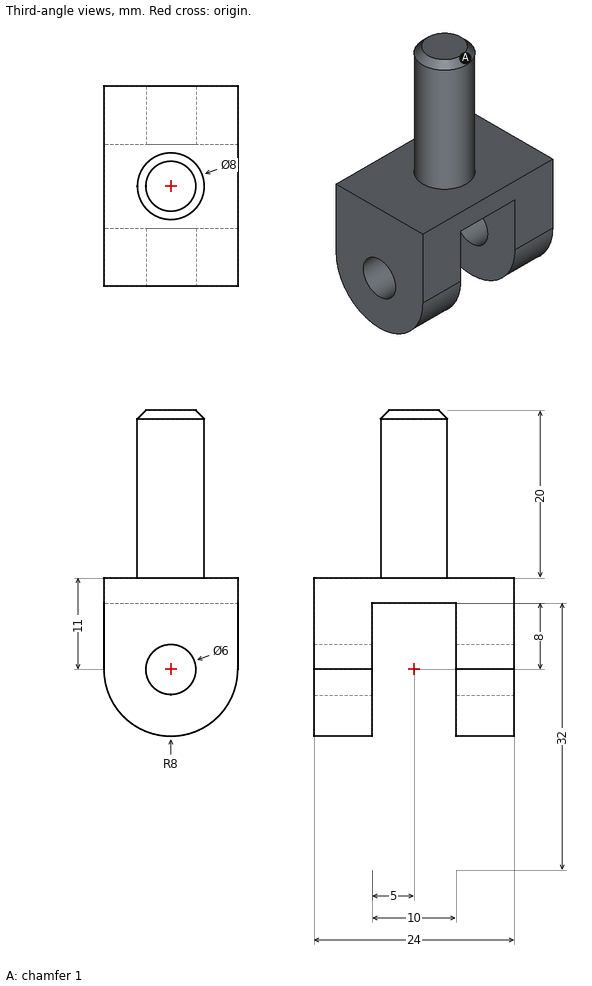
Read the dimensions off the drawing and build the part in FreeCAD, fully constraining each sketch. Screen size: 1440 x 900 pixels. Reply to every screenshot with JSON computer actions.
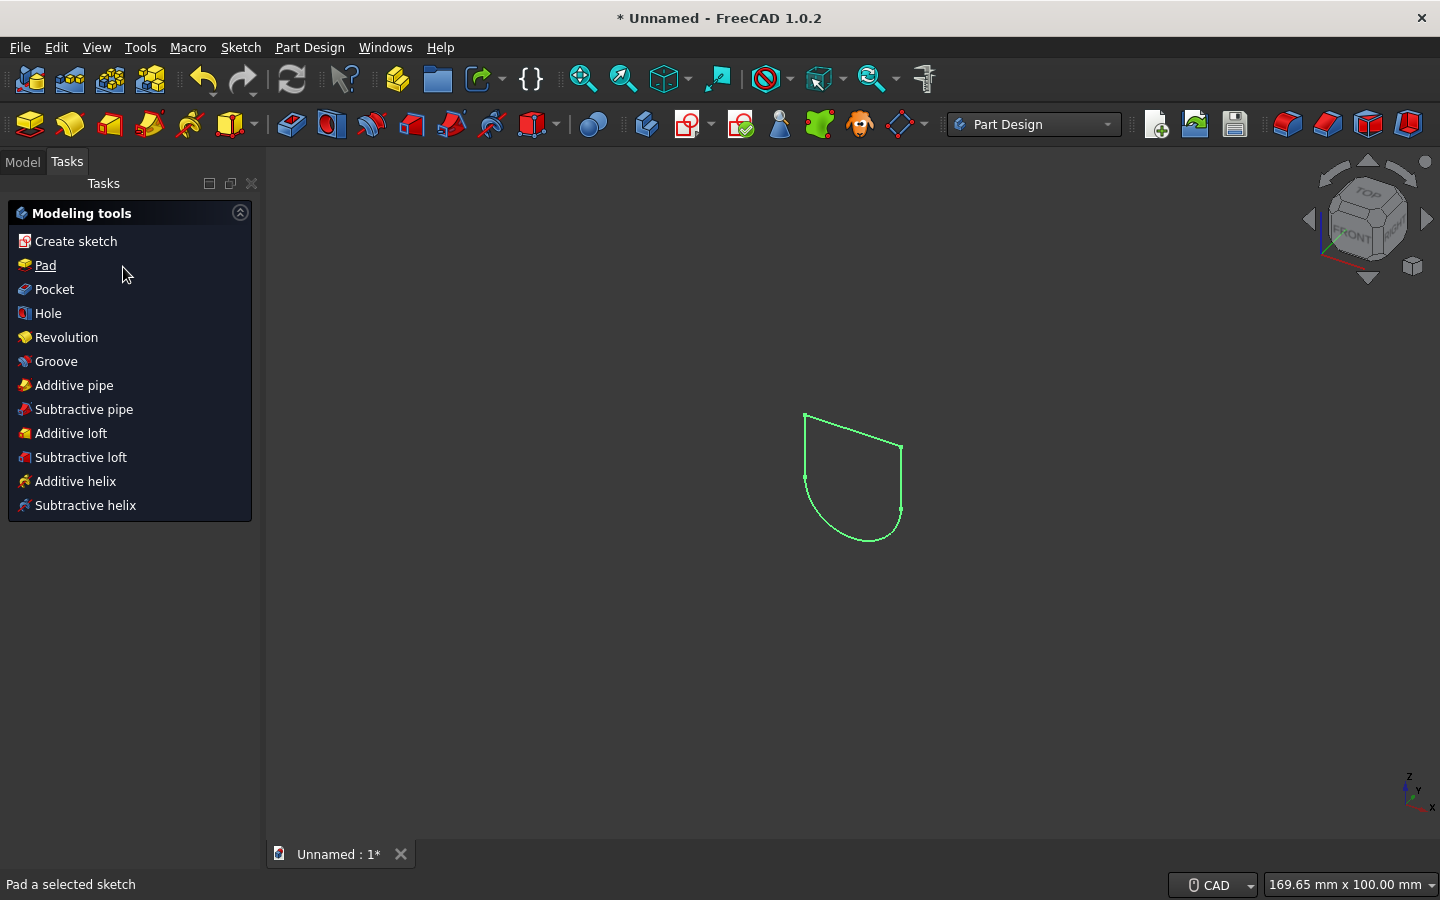
{"action": "left_click", "coordinate": [30, 124]}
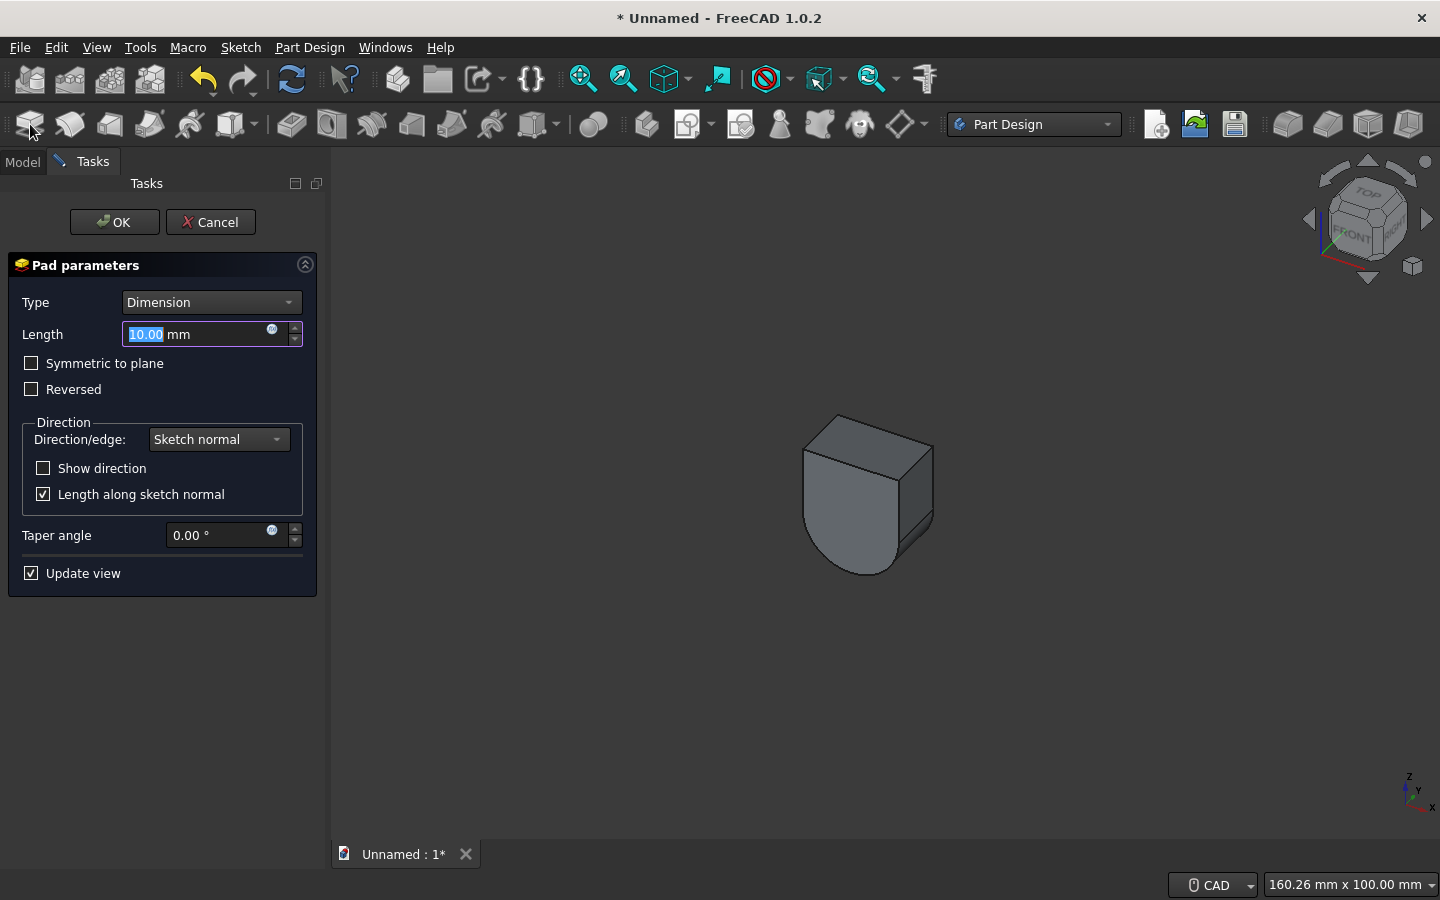
{"action": "type", "text": "24"}
{"action": "key", "text": "Tab"}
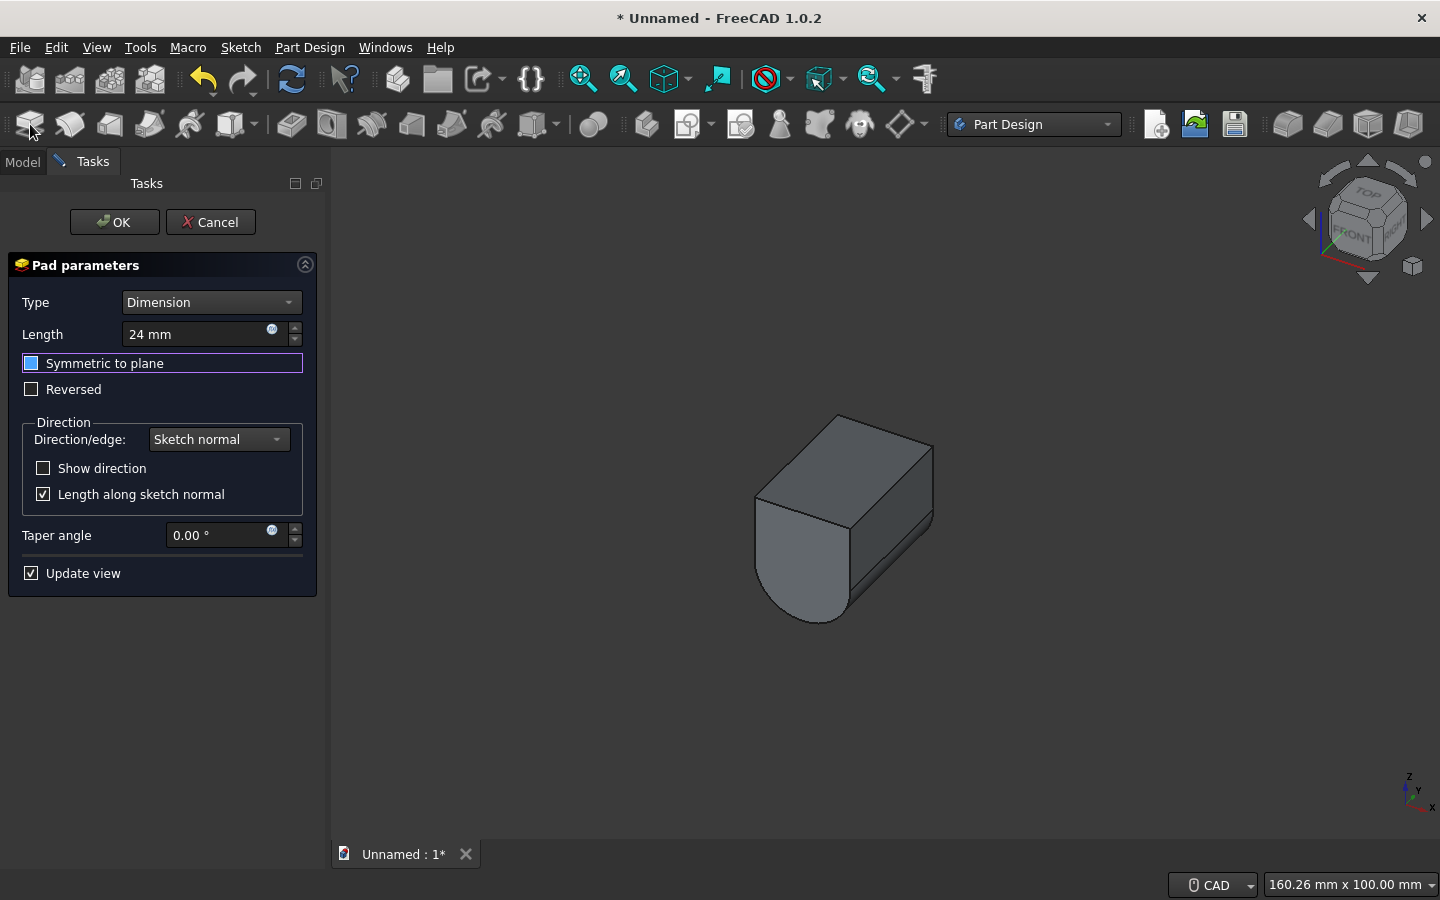
{"action": "left_click", "coordinate": [30, 363]}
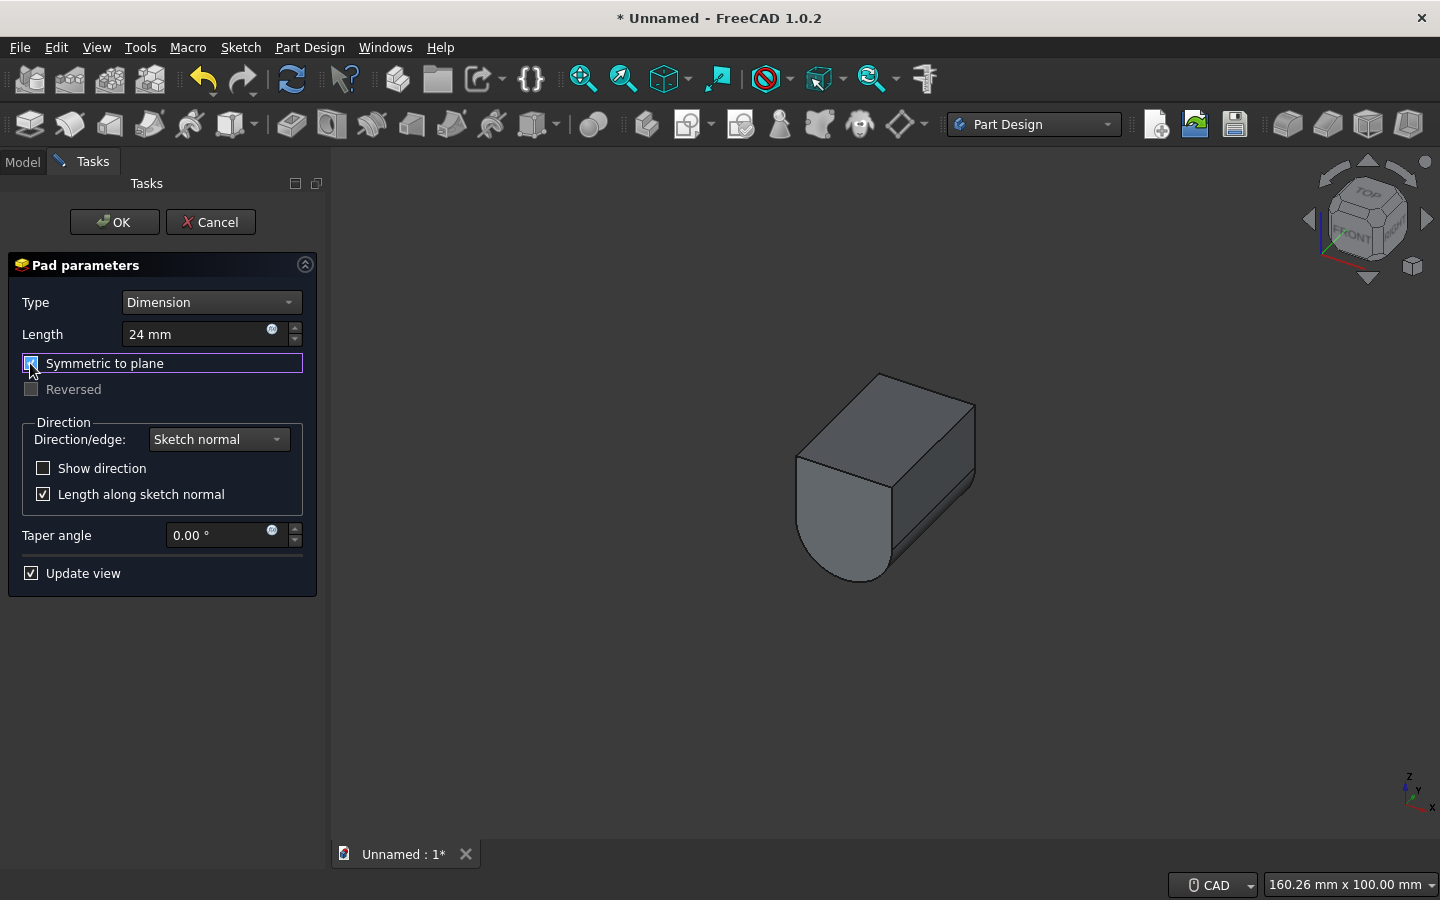
{"action": "left_click", "coordinate": [115, 222]}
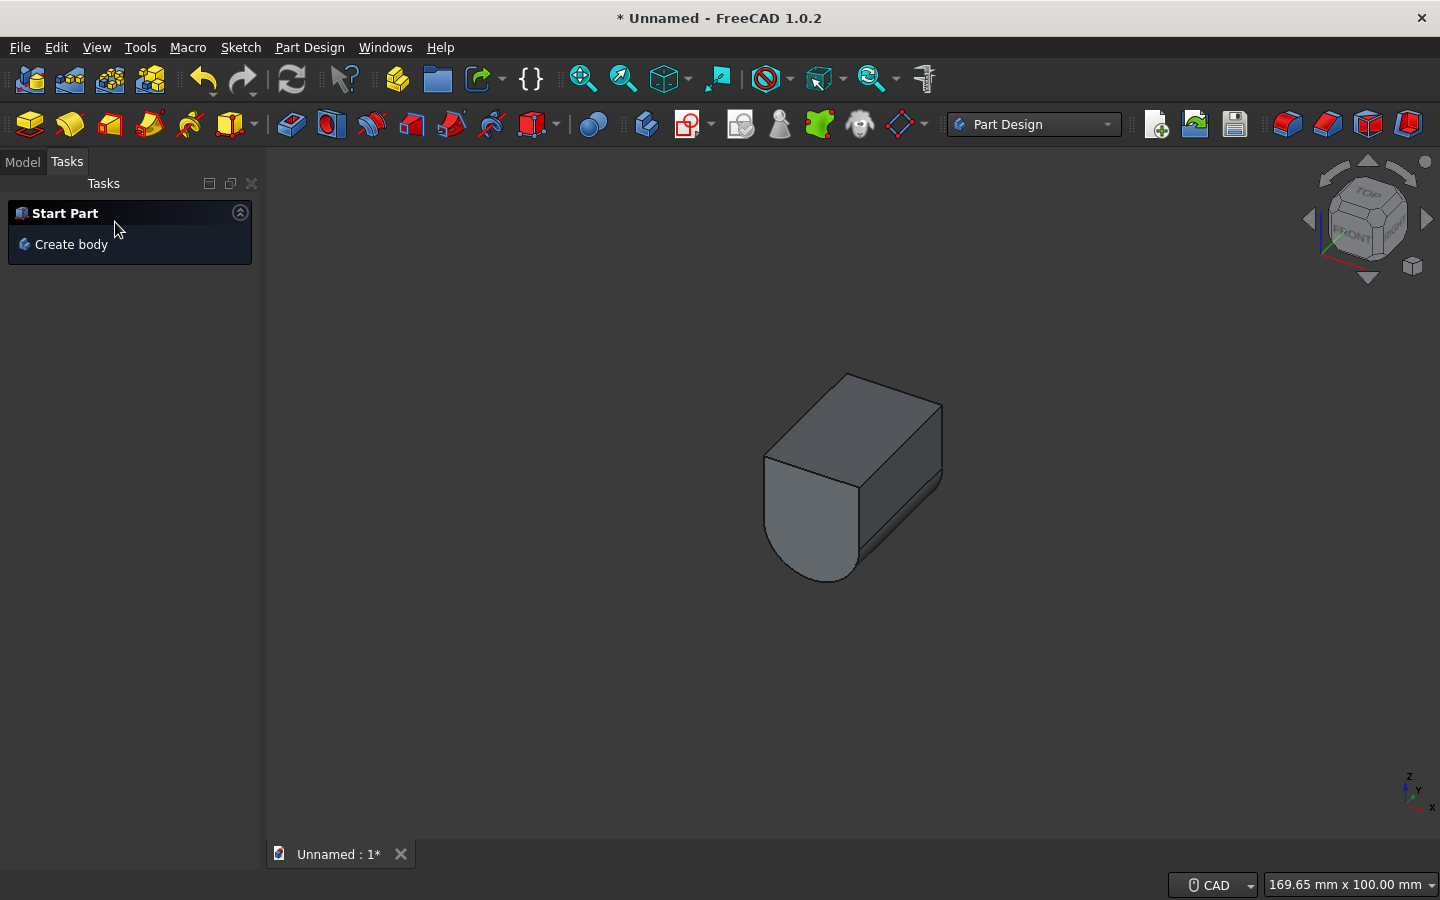
{"action": "left_click", "coordinate": [584, 80]}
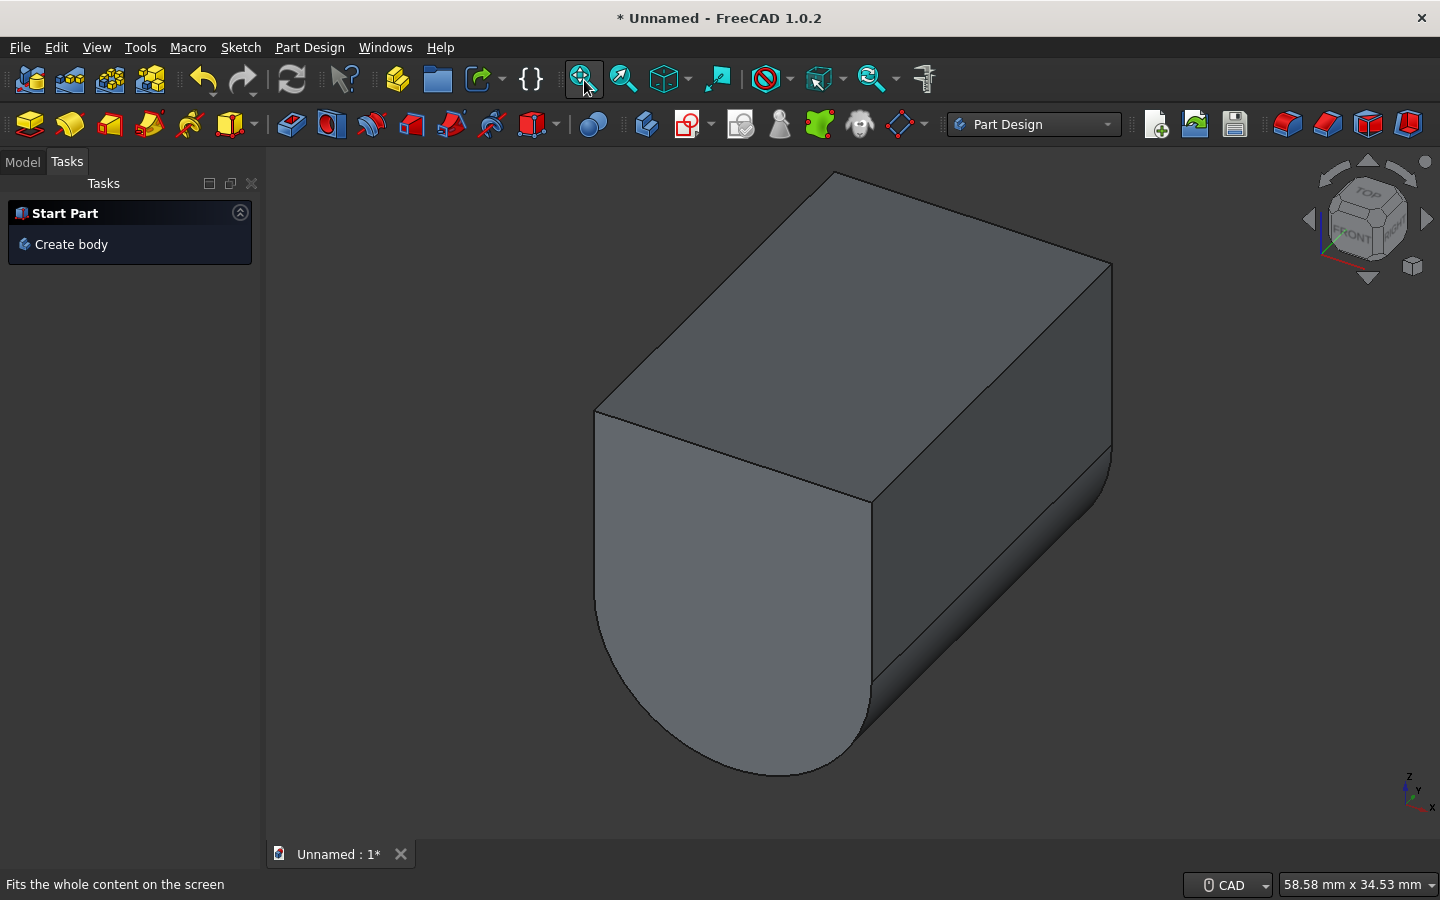
{"action": "left_click", "coordinate": [887, 302]}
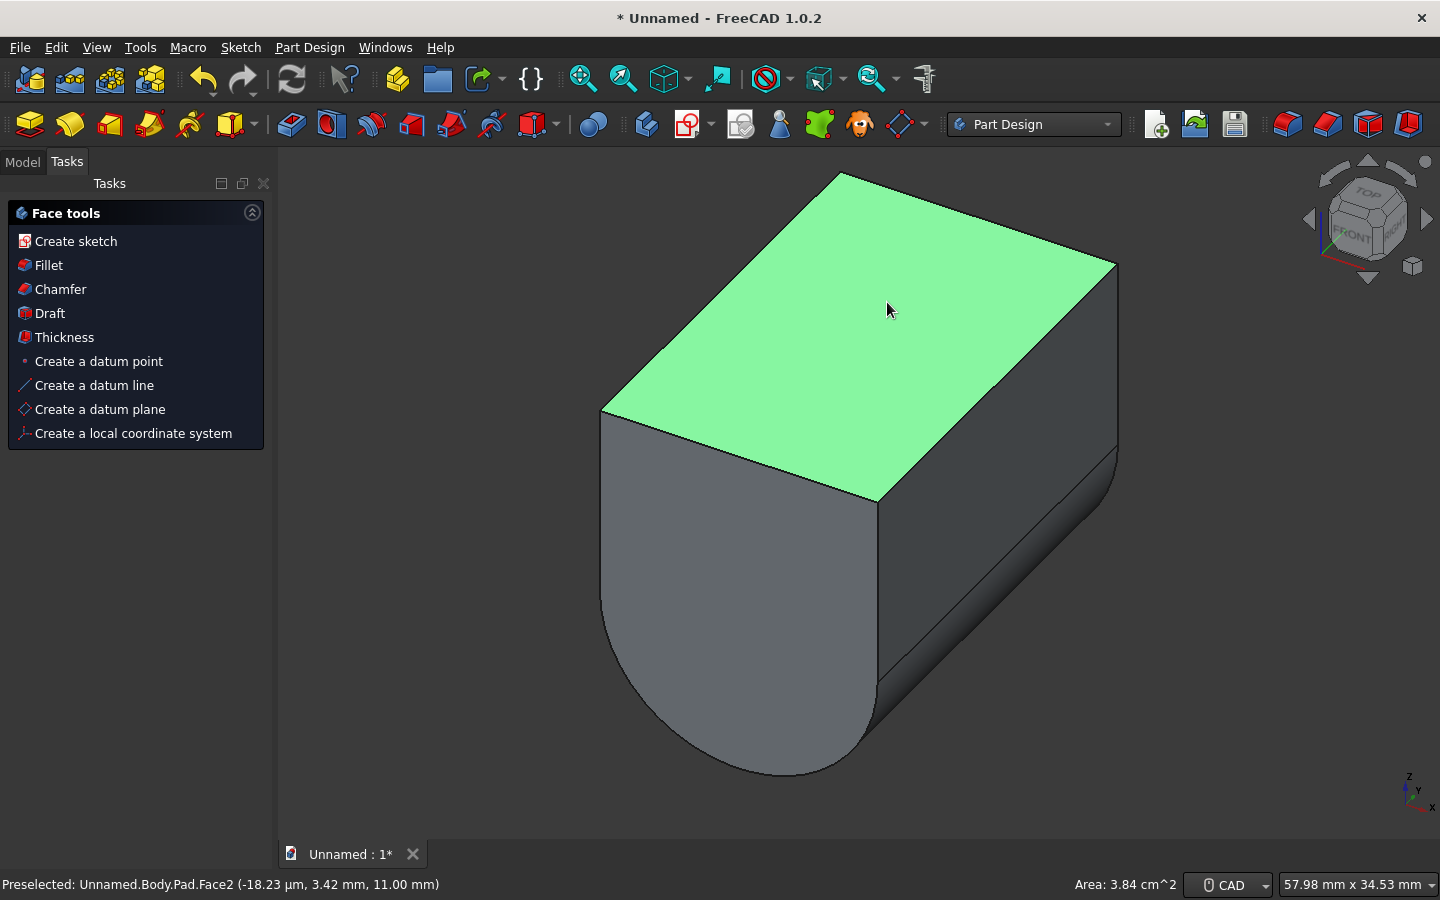
{"action": "left_click", "coordinate": [688, 124]}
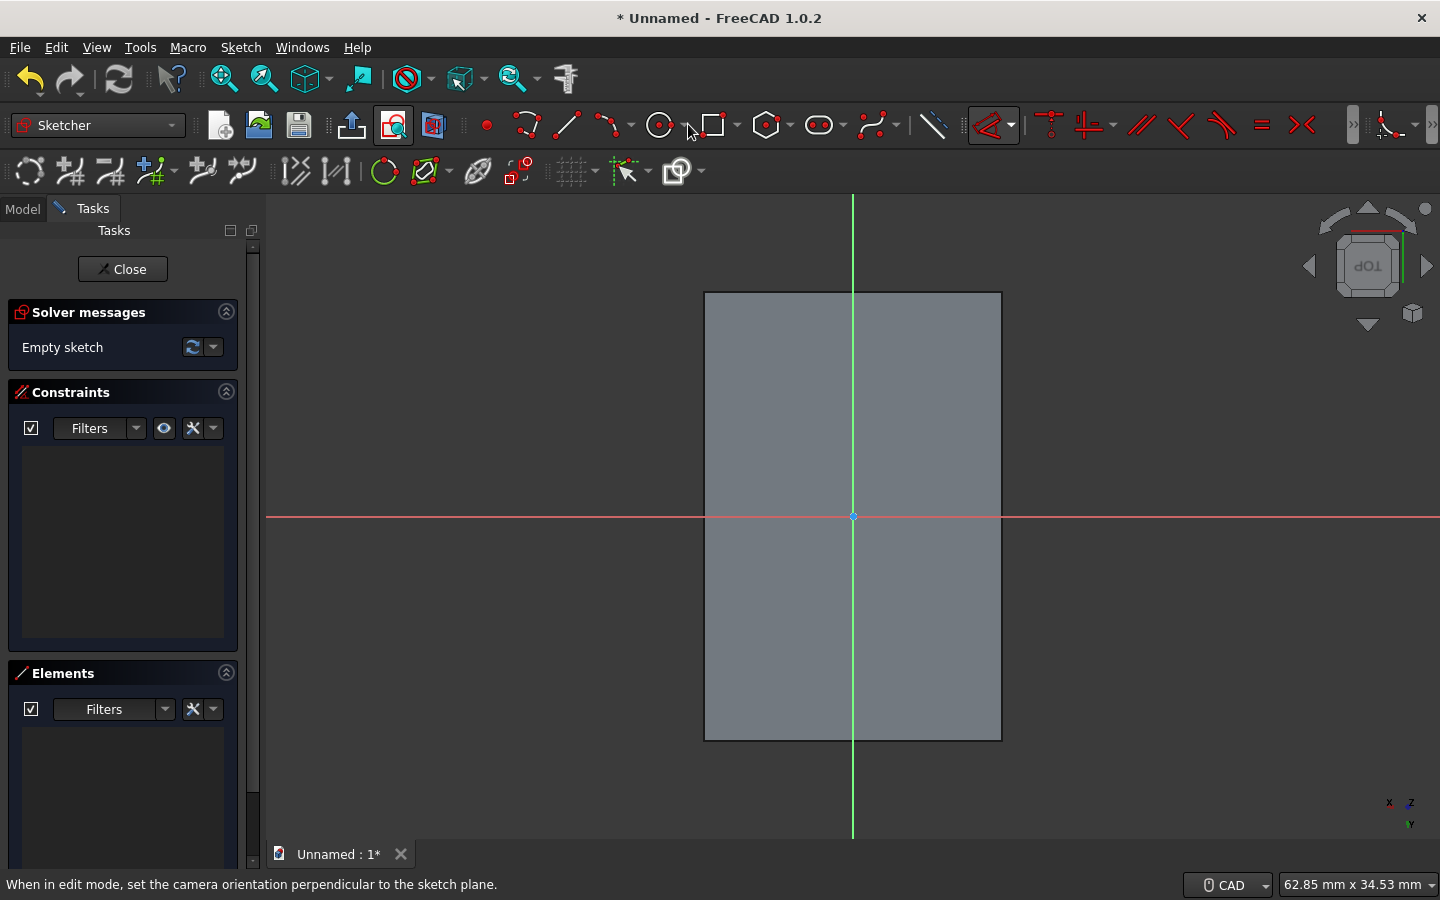
{"action": "scroll", "coordinate": [893, 516], "scroll_direction": "up", "scroll_amount": 5}